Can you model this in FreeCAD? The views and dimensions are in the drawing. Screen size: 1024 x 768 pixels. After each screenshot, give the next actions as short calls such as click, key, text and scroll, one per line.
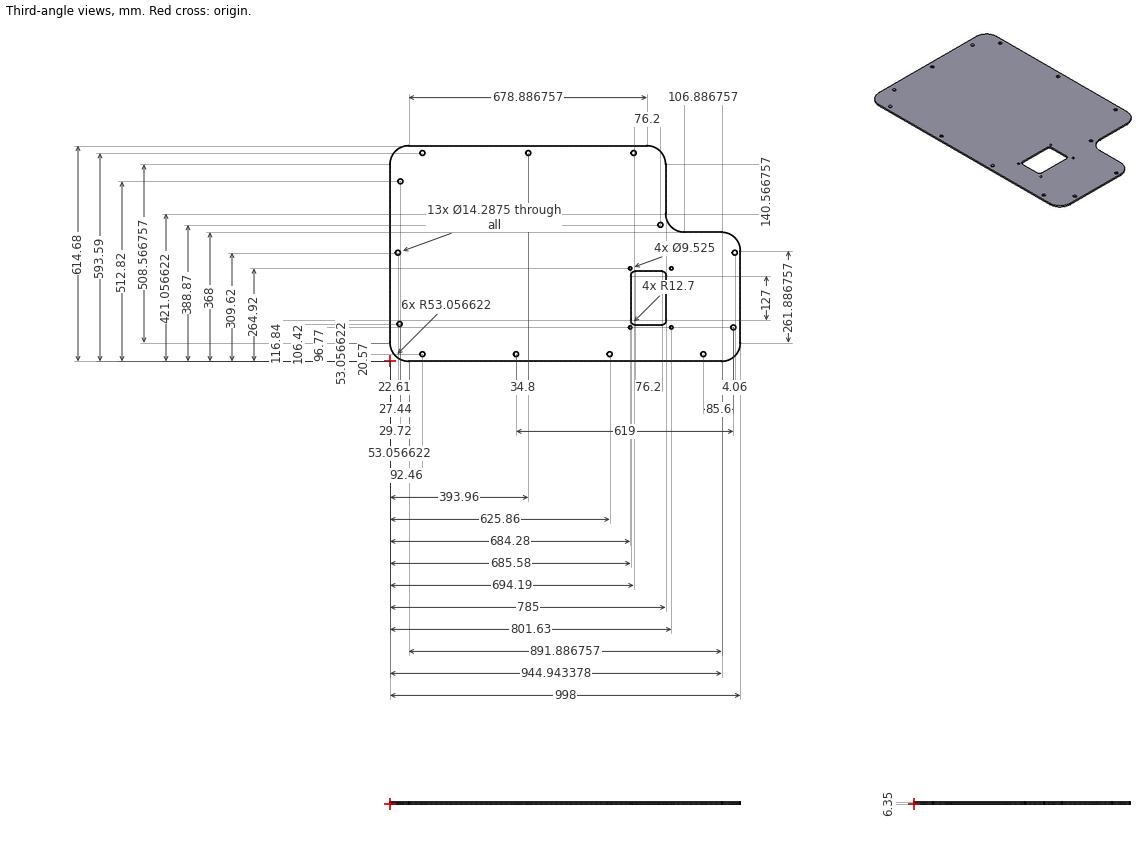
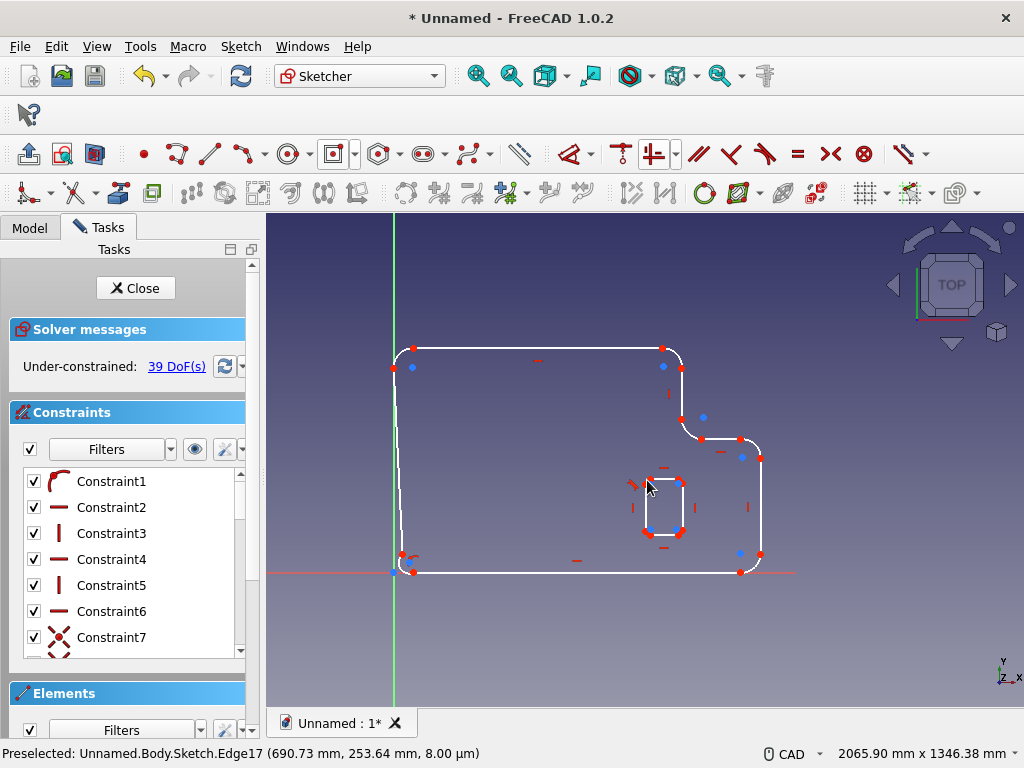
click(646, 517)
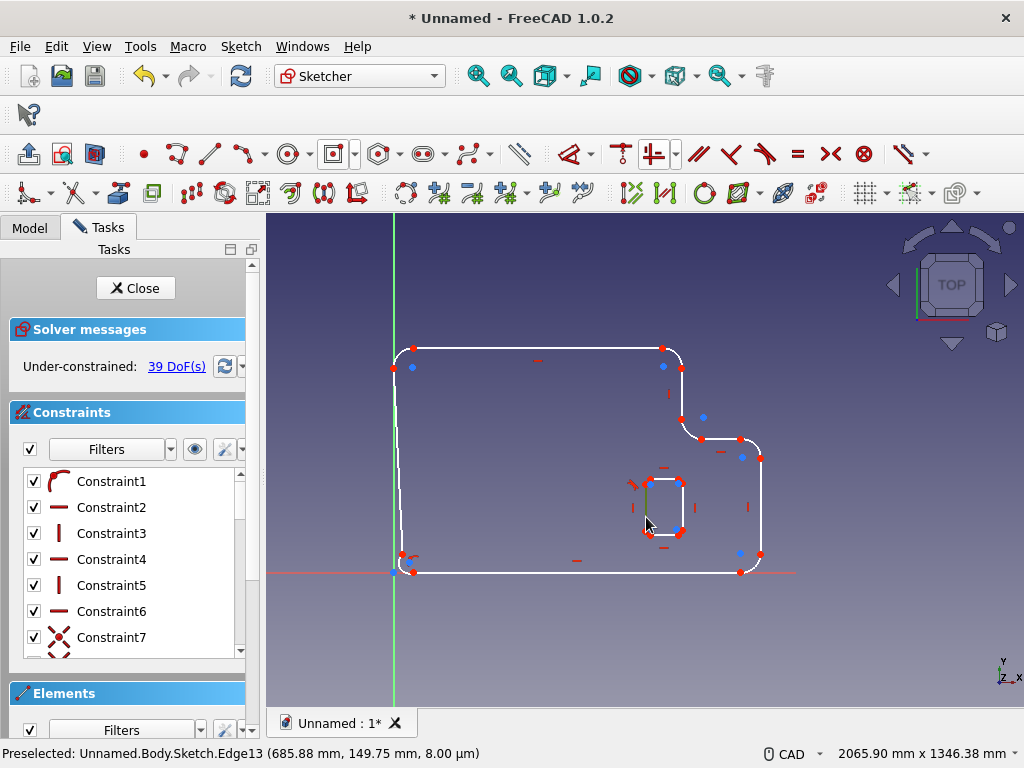
scroll(647, 534, up, 8)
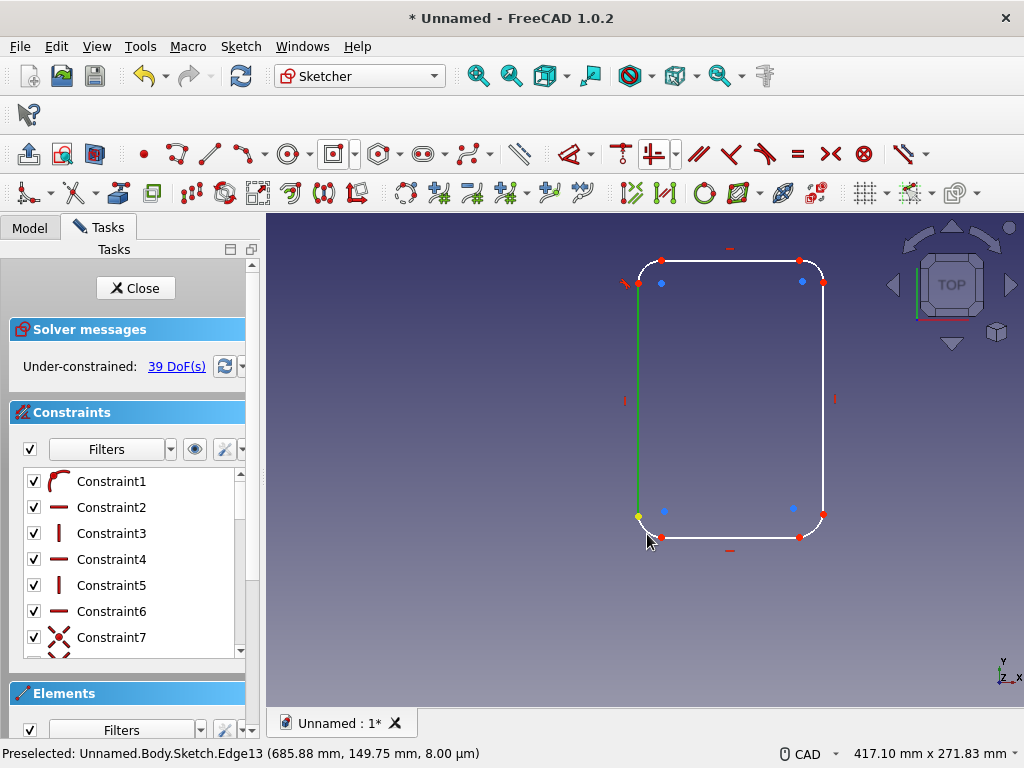
click(646, 531)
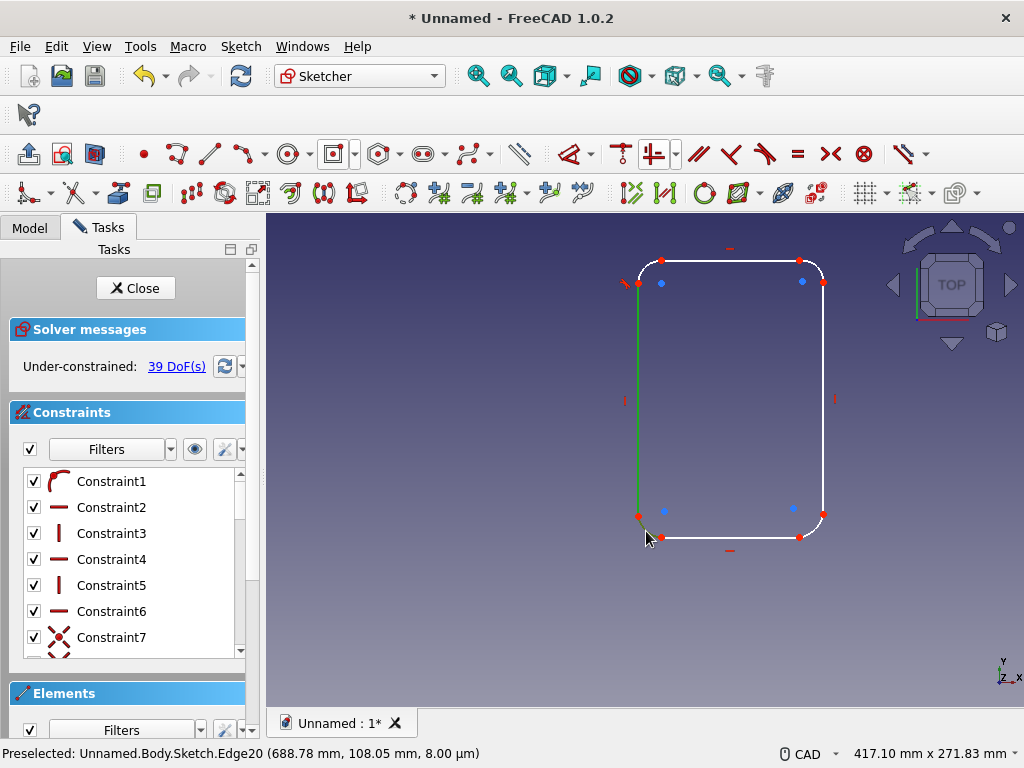
click(765, 154)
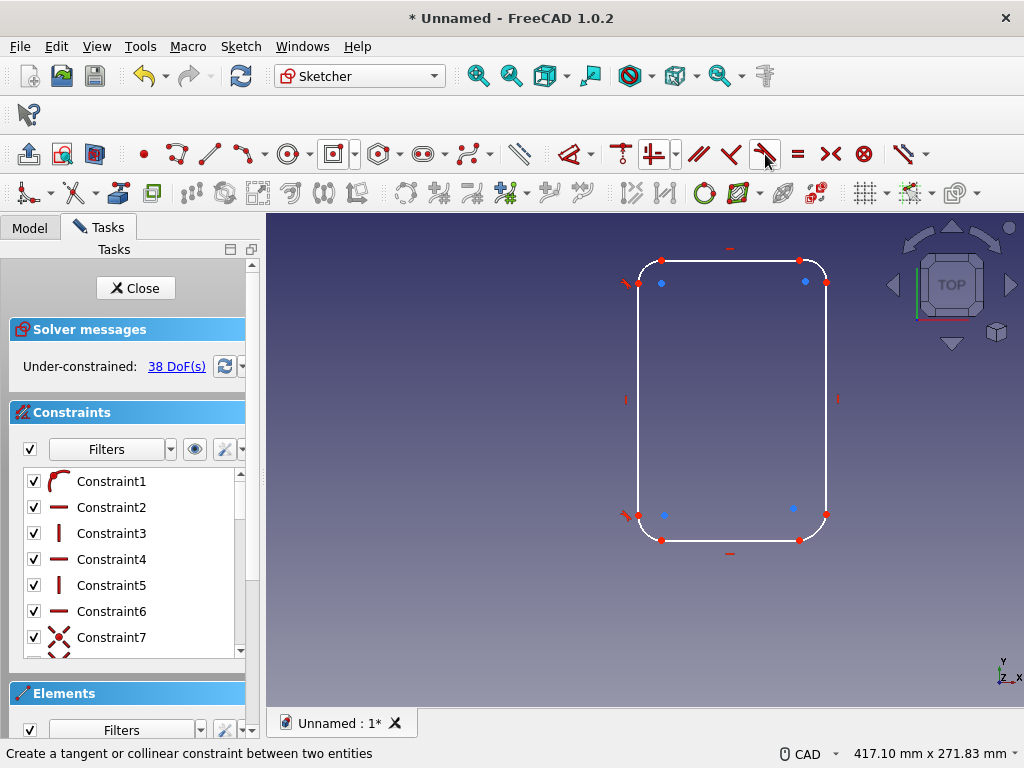
scroll(647, 534, down, 8)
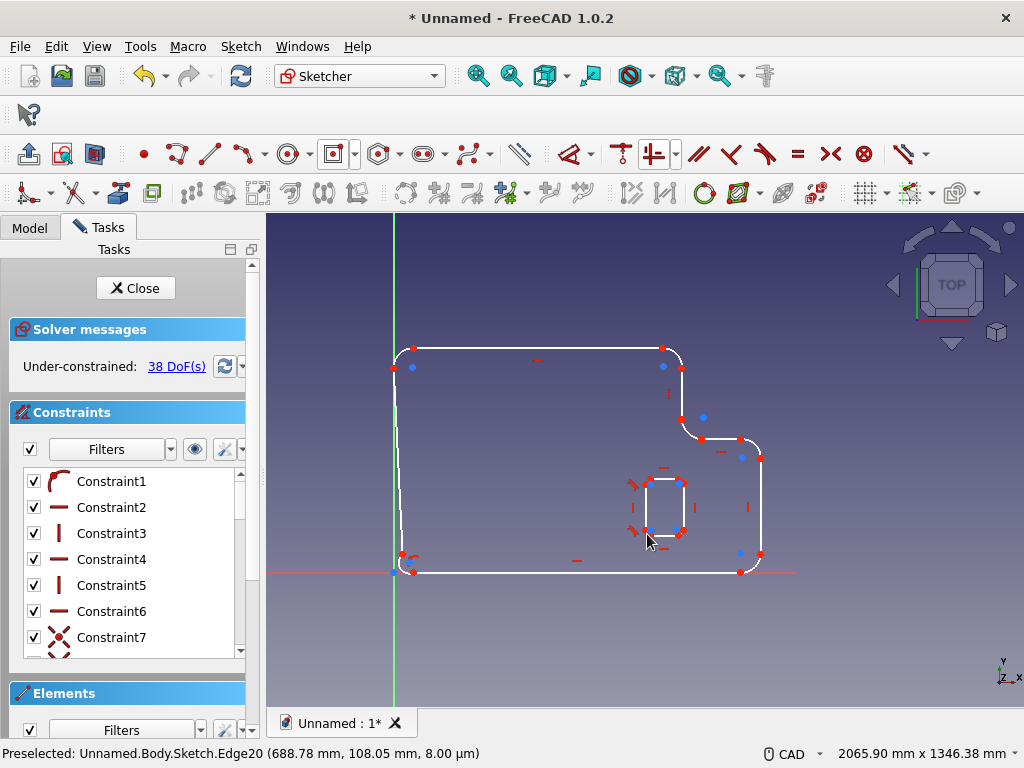
scroll(659, 479, up, 3)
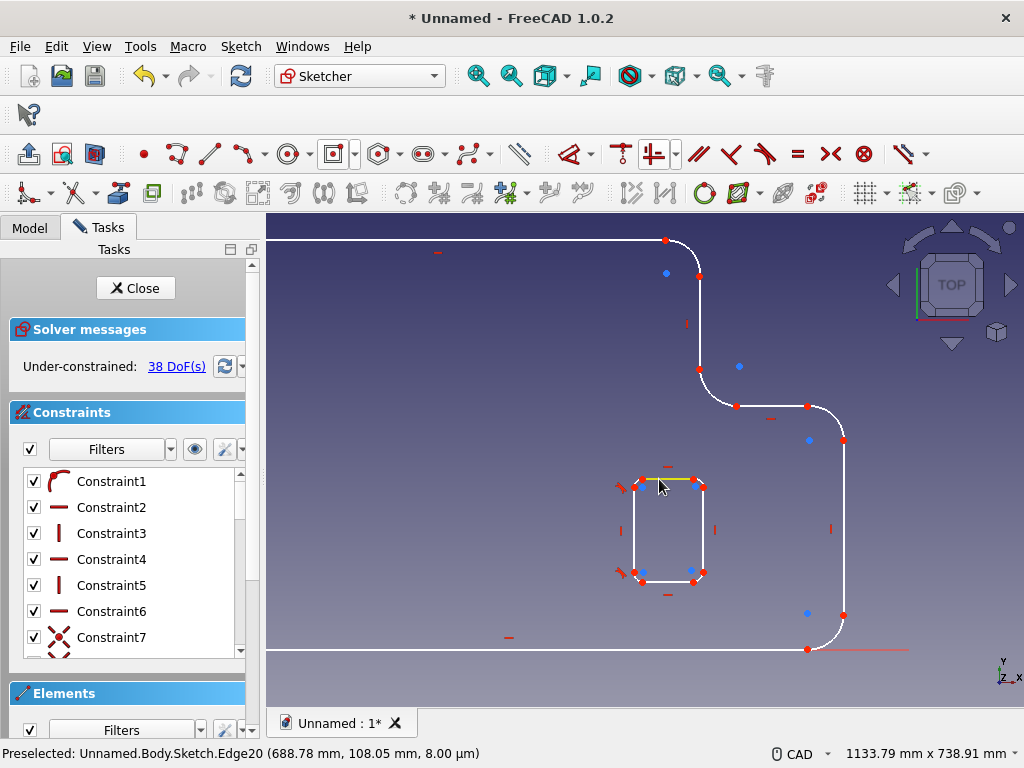
click(658, 479)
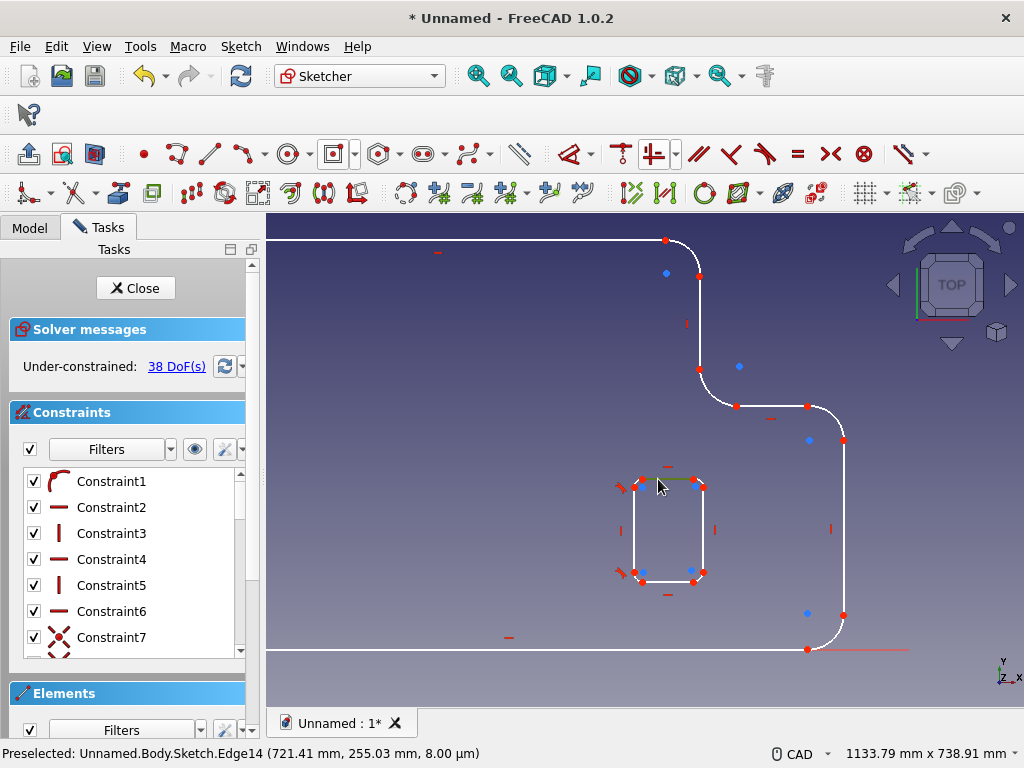
scroll(637, 482, up, 4)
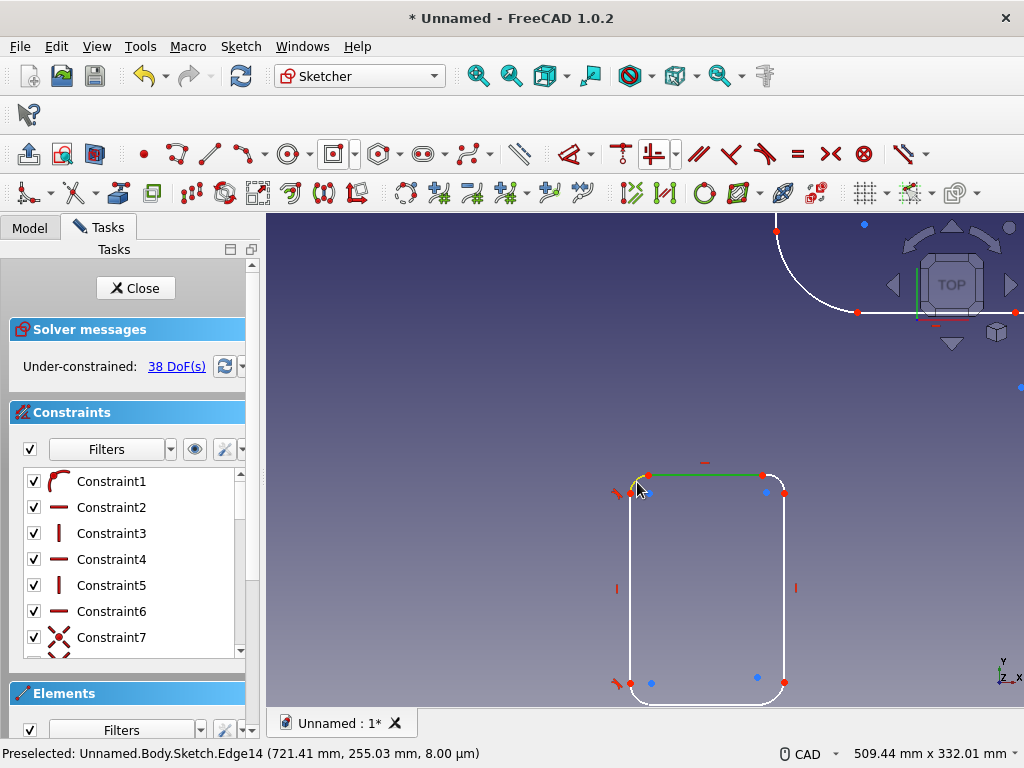
click(636, 481)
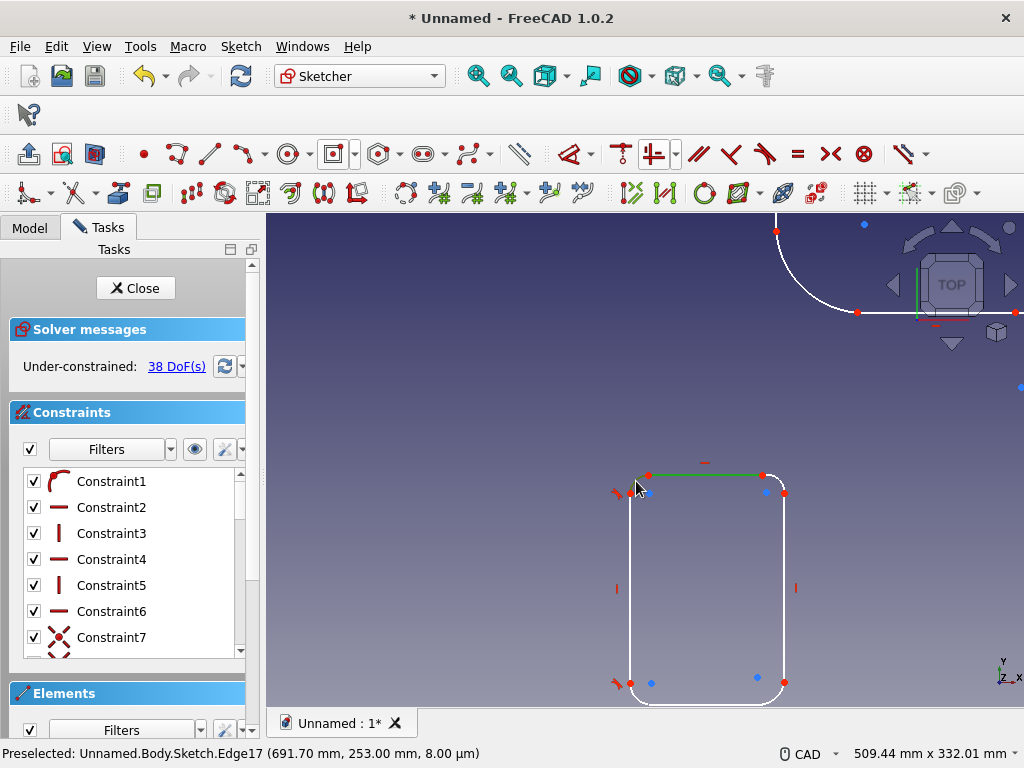
click(765, 154)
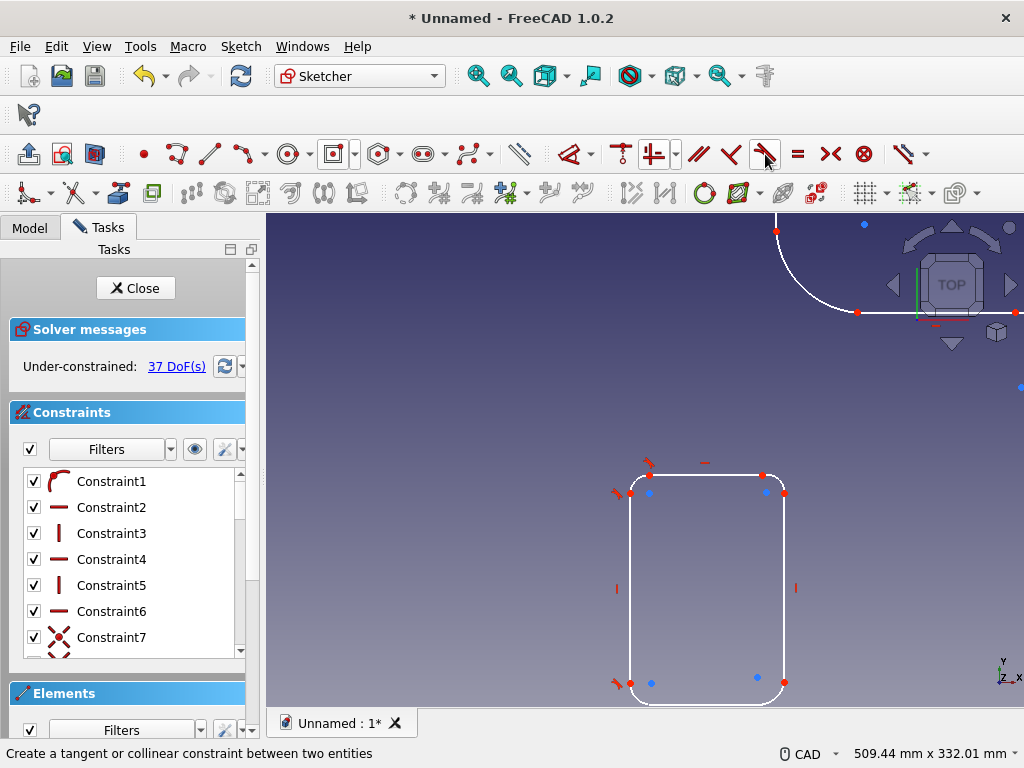
click(683, 475)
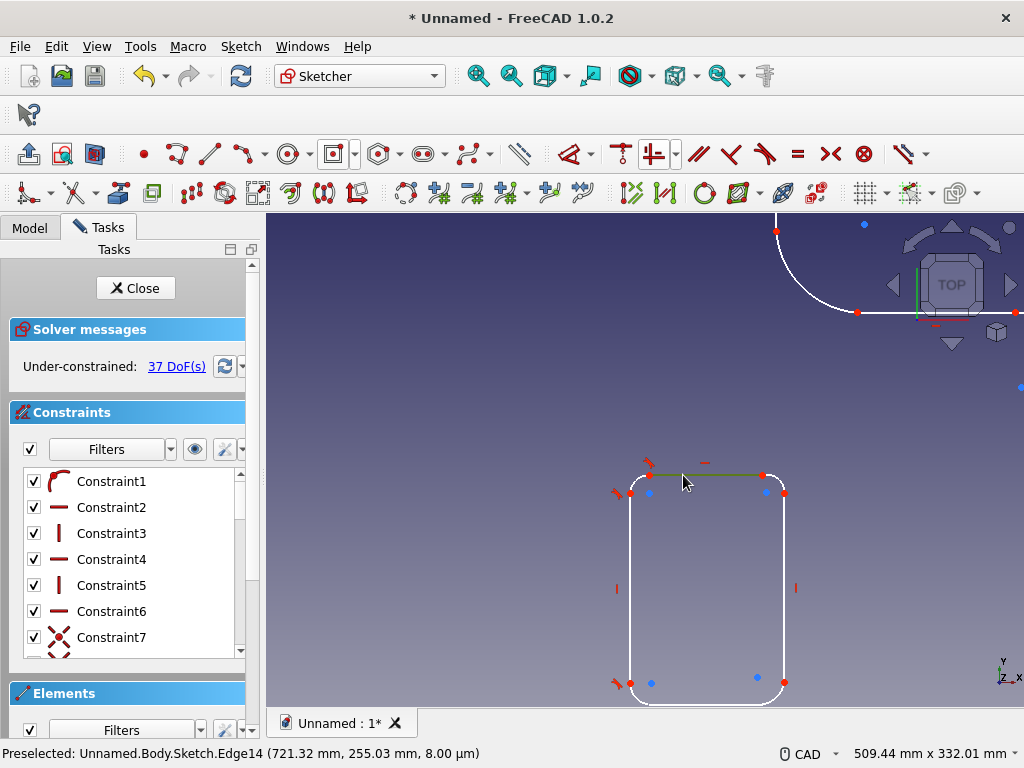
scroll(782, 484, up, 2)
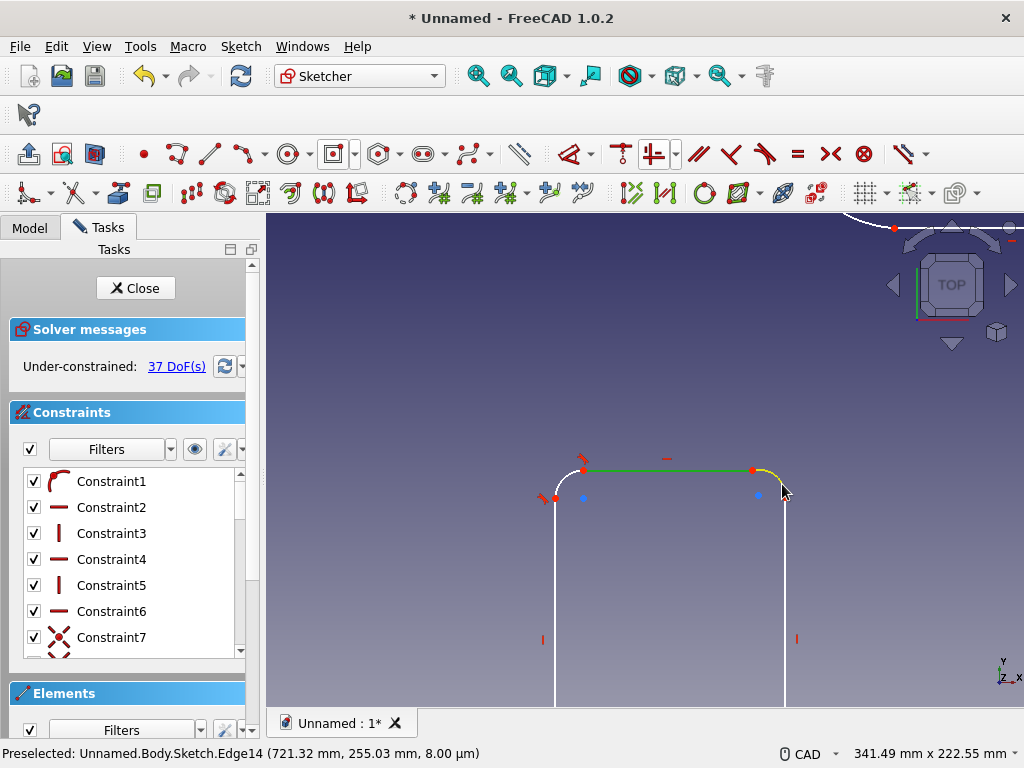
click(782, 483)